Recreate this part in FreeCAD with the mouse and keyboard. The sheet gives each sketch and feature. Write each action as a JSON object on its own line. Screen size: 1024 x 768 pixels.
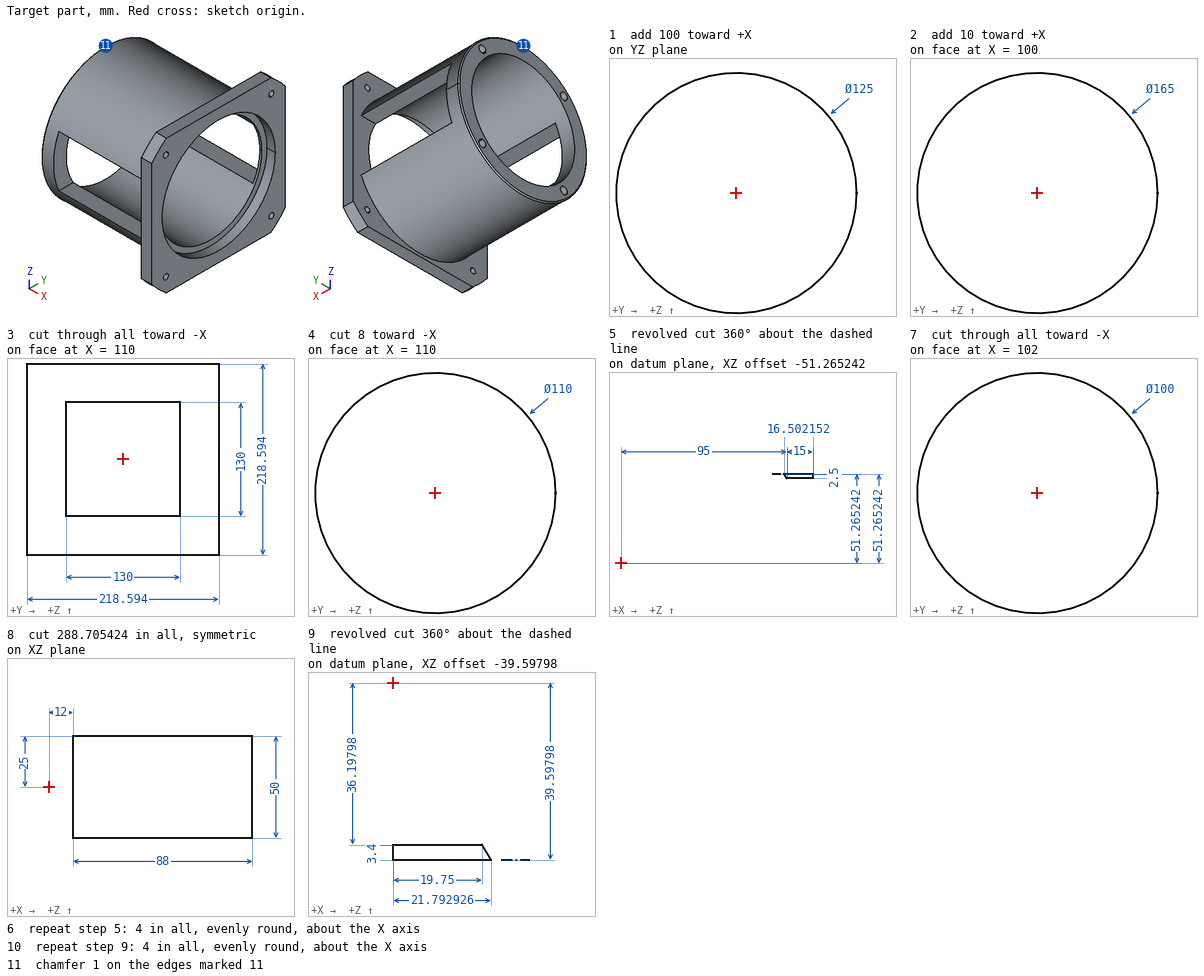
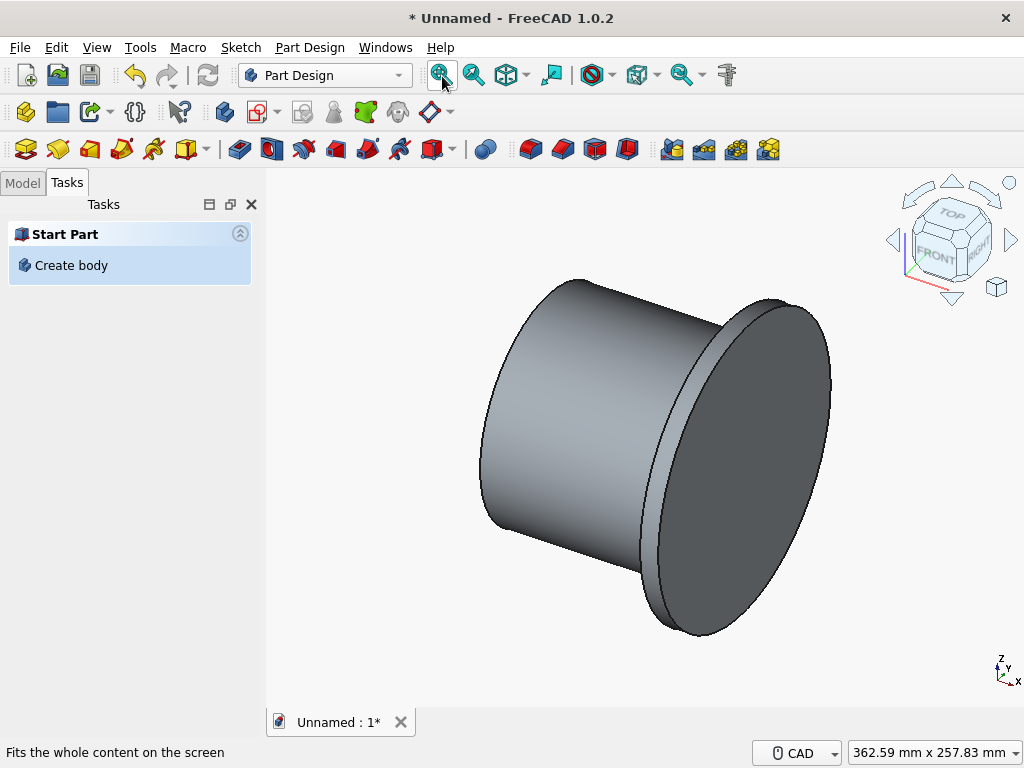
{"action": "left_click", "coordinate": [744, 470]}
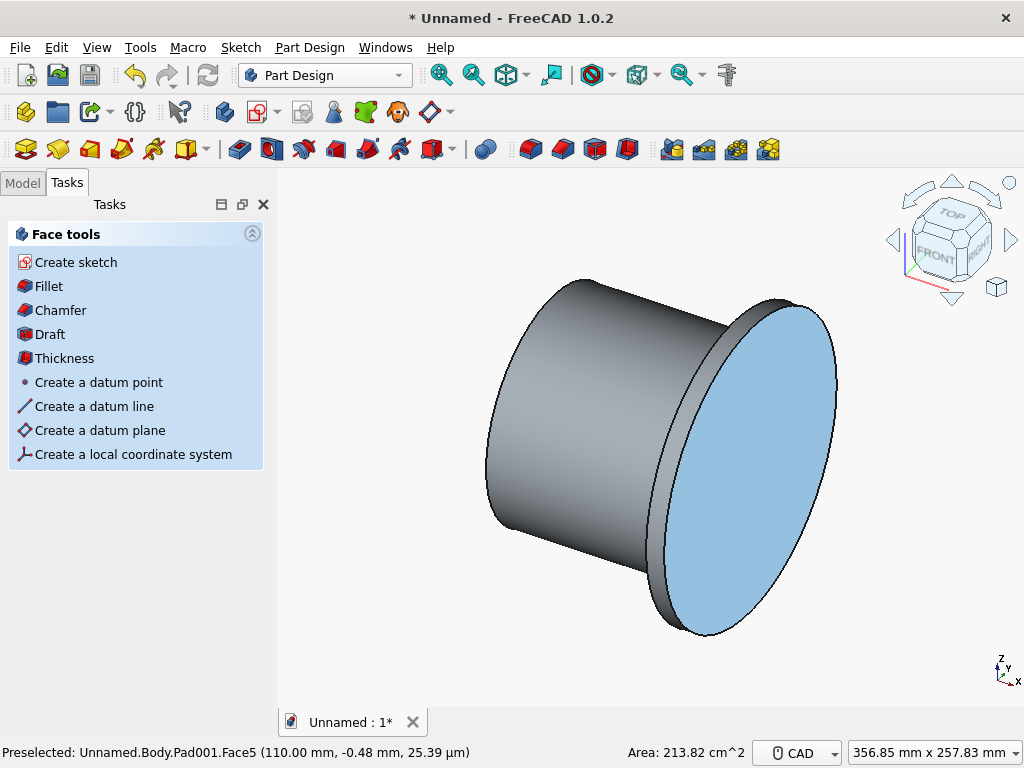
{"action": "left_click", "coordinate": [258, 112]}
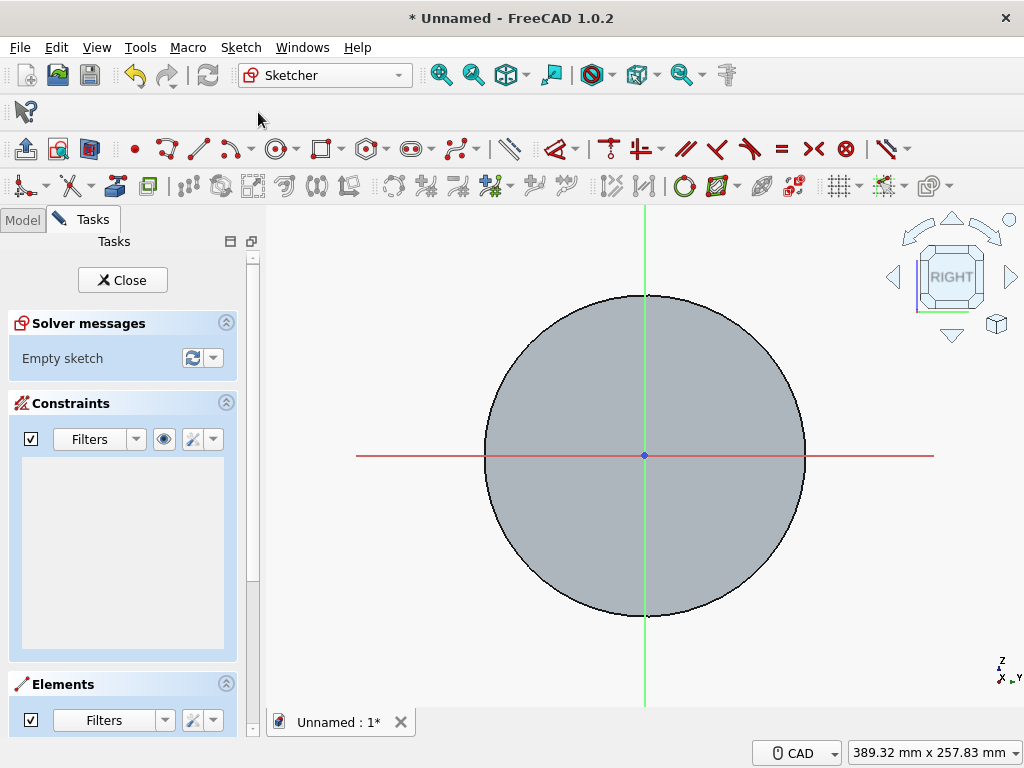
{"action": "scroll", "coordinate": [438, 456], "scroll_direction": "down", "scroll_amount": 2}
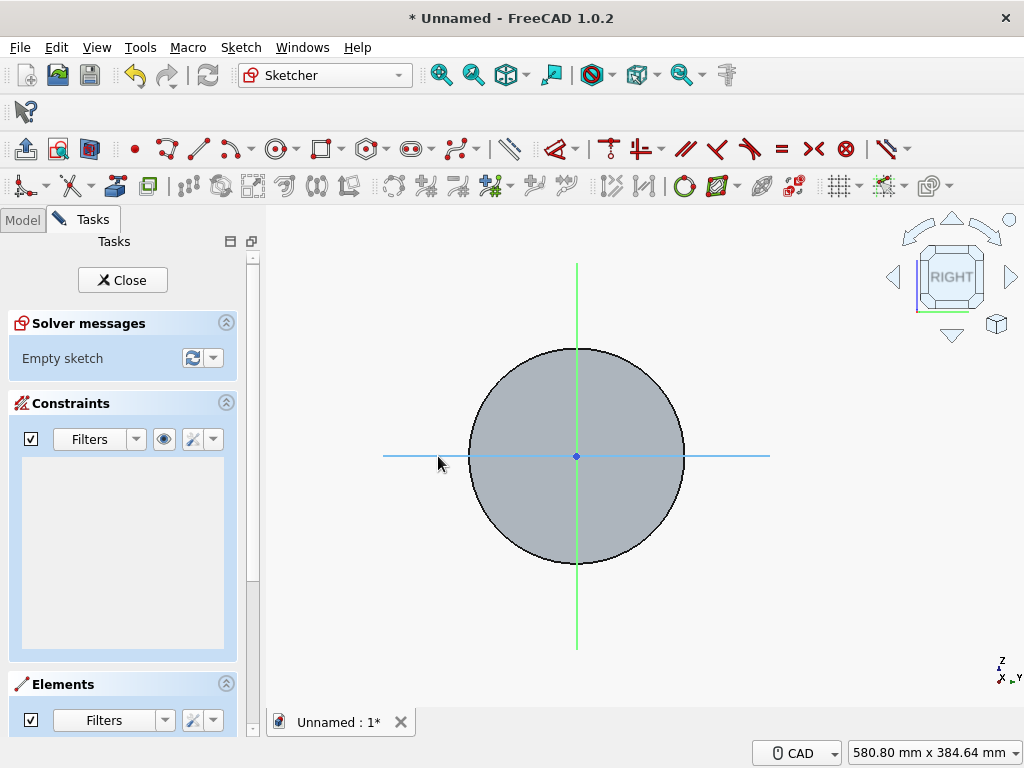
{"action": "left_click", "coordinate": [344, 150]}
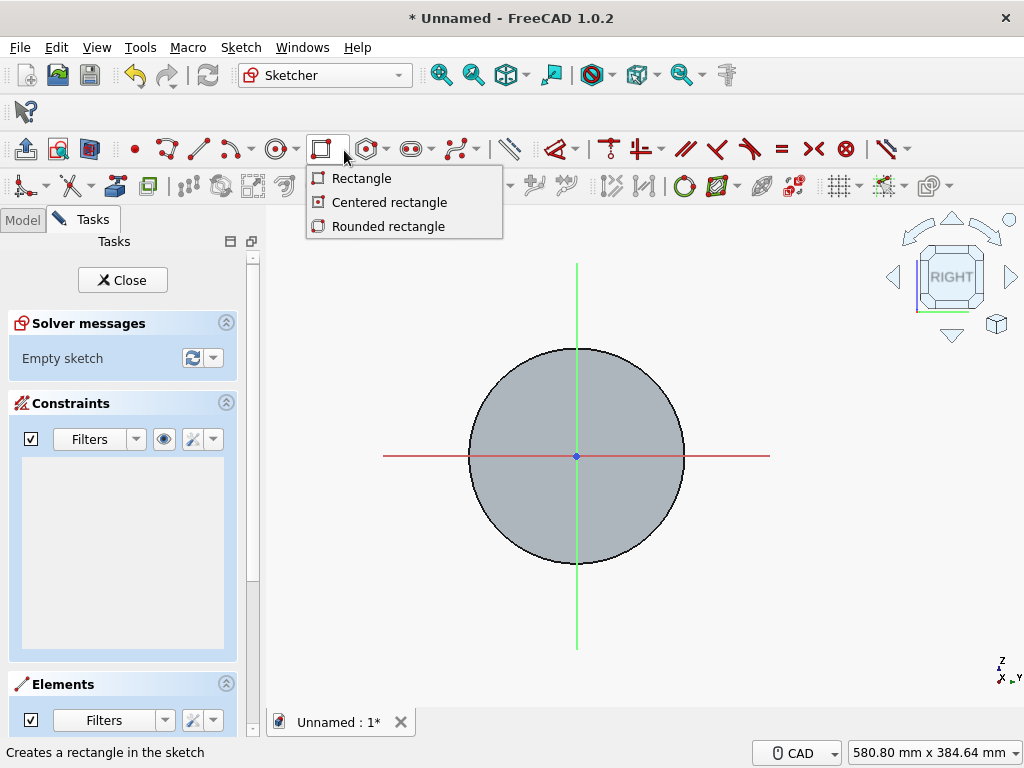
{"action": "left_click", "coordinate": [404, 202]}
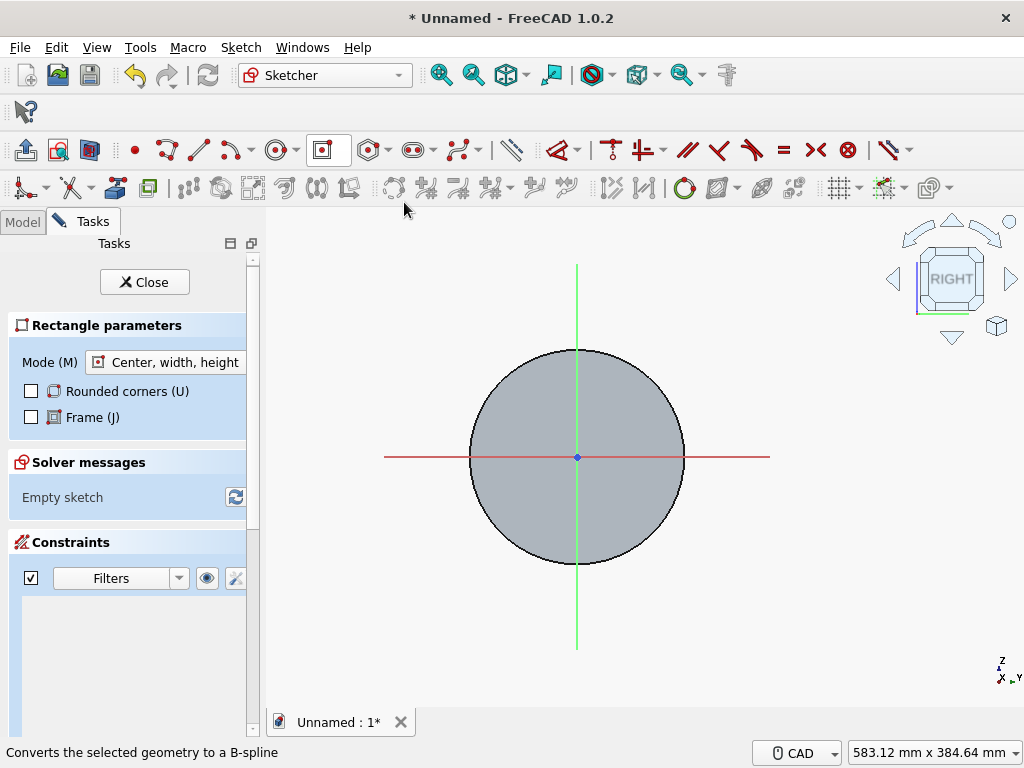
{"action": "left_click", "coordinate": [577, 457]}
{"action": "mouse_move", "coordinate": [719, 315]}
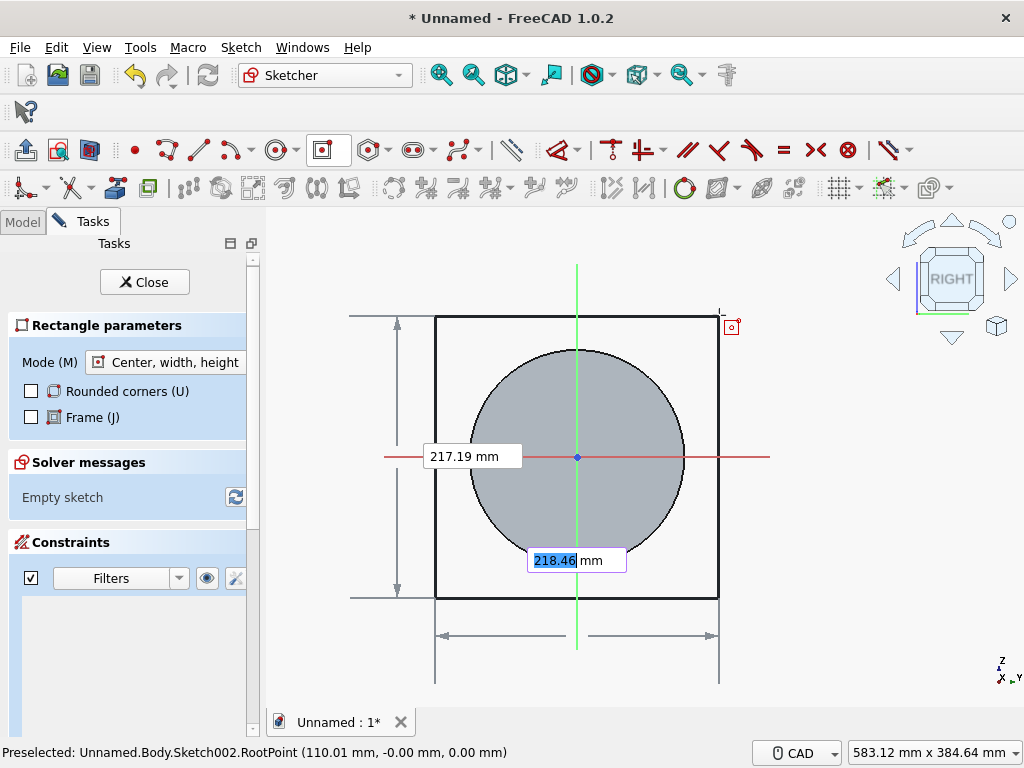
{"action": "type", "text": "218.594"}
{"action": "key", "text": "Tab"}
{"action": "type", "text": "218.594"}
{"action": "key", "text": "Return"}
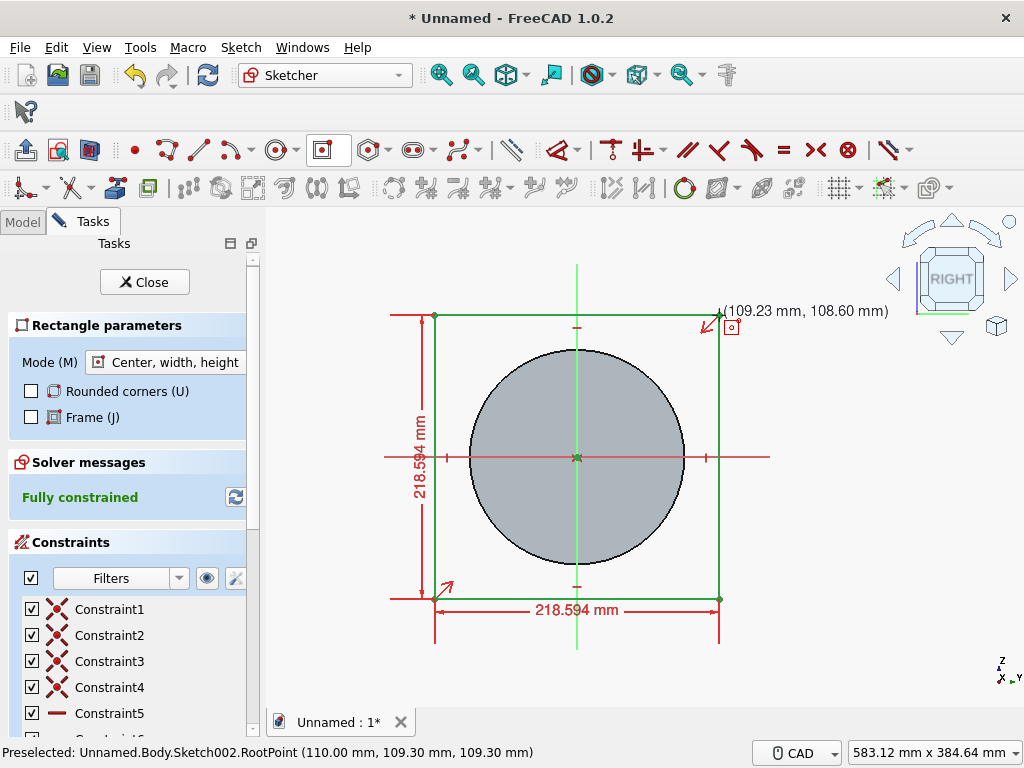
{"action": "left_click", "coordinate": [577, 457]}
{"action": "mouse_move", "coordinate": [662, 373]}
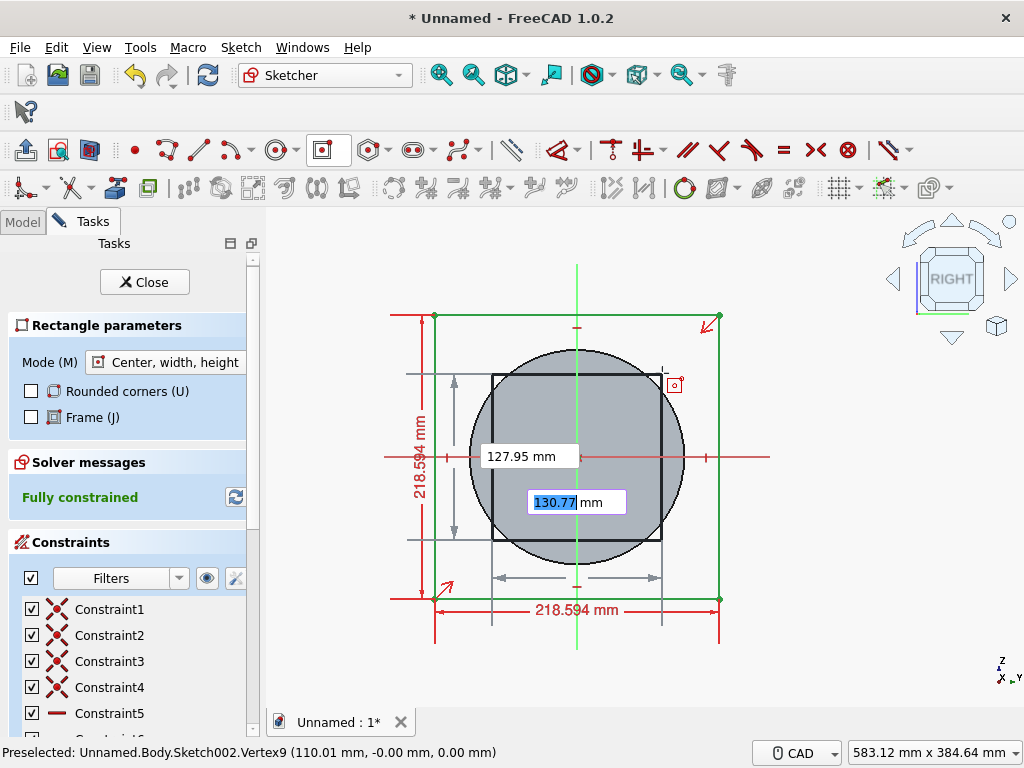
{"action": "type", "text": "130"}
{"action": "key", "text": "Tab"}
{"action": "type", "text": "130"}
{"action": "key", "text": "Return"}
{"action": "key", "text": "Escape"}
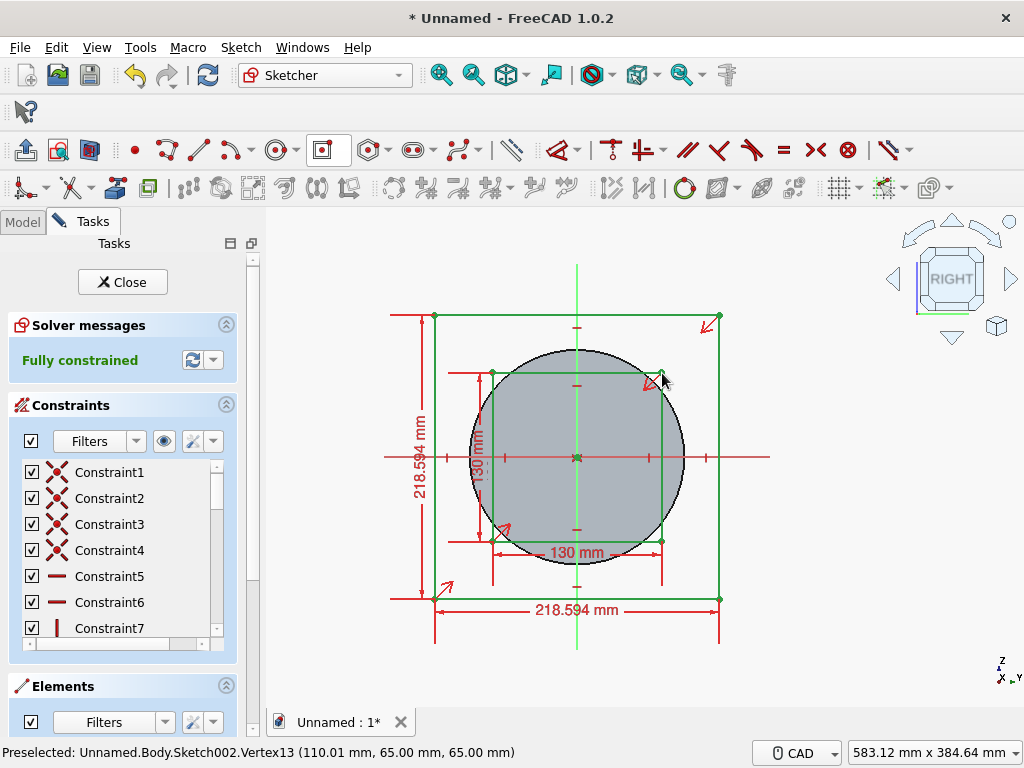
{"action": "left_click", "coordinate": [123, 282]}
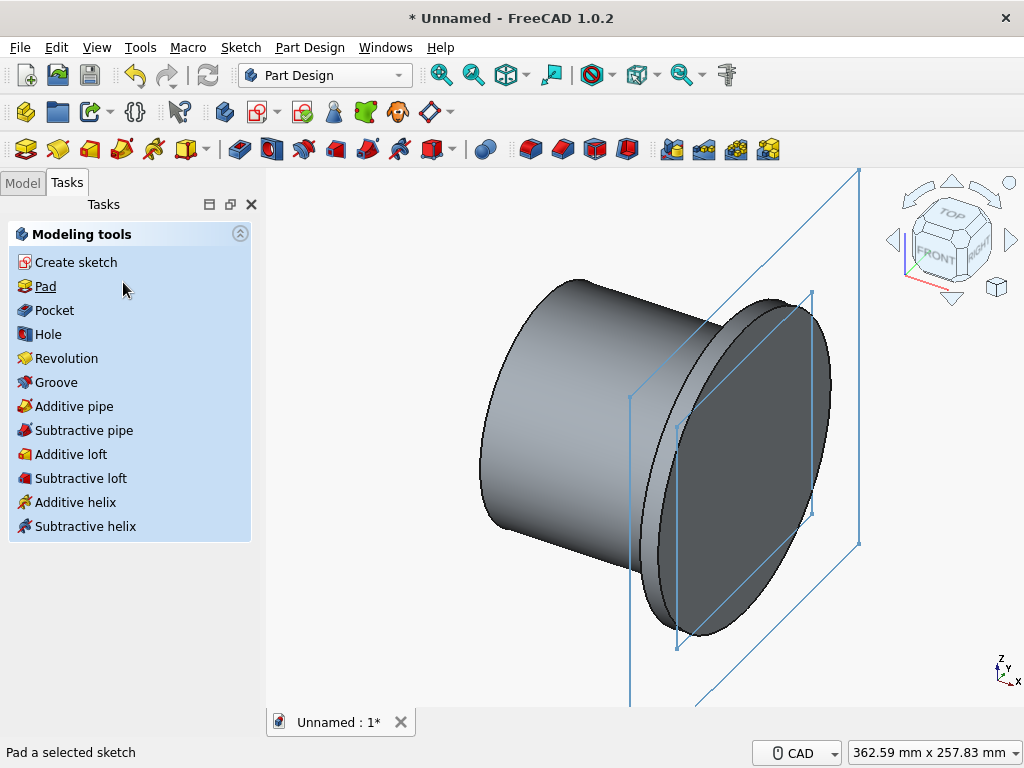
{"action": "left_click", "coordinate": [240, 150]}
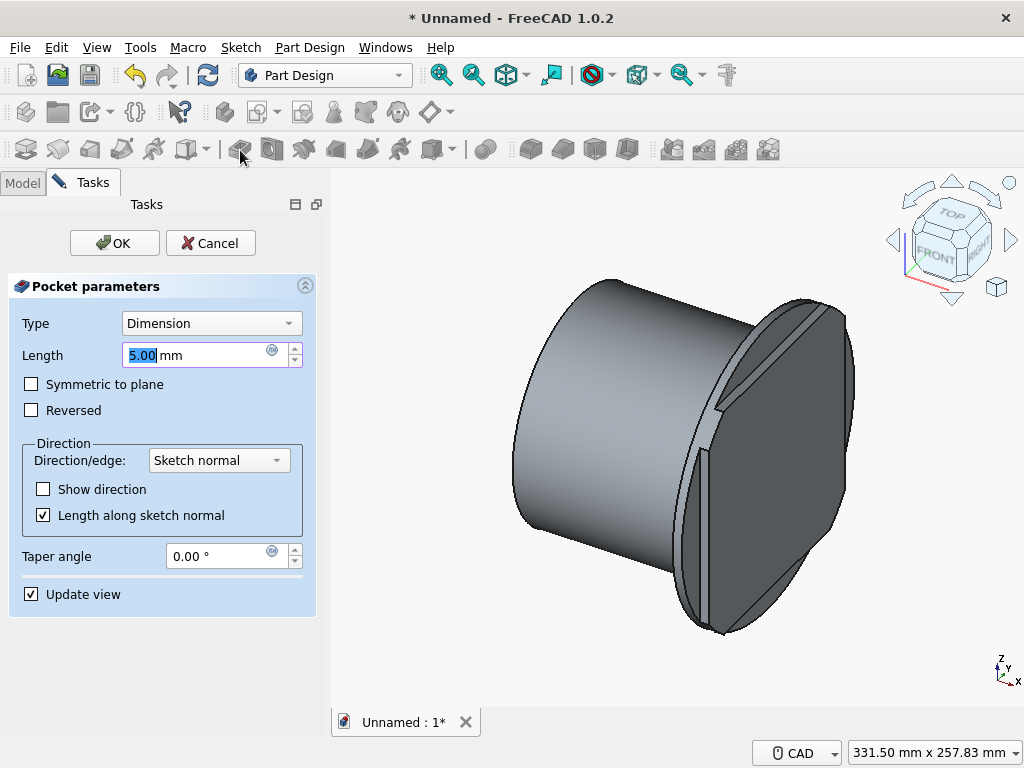
{"action": "left_click", "coordinate": [212, 324]}